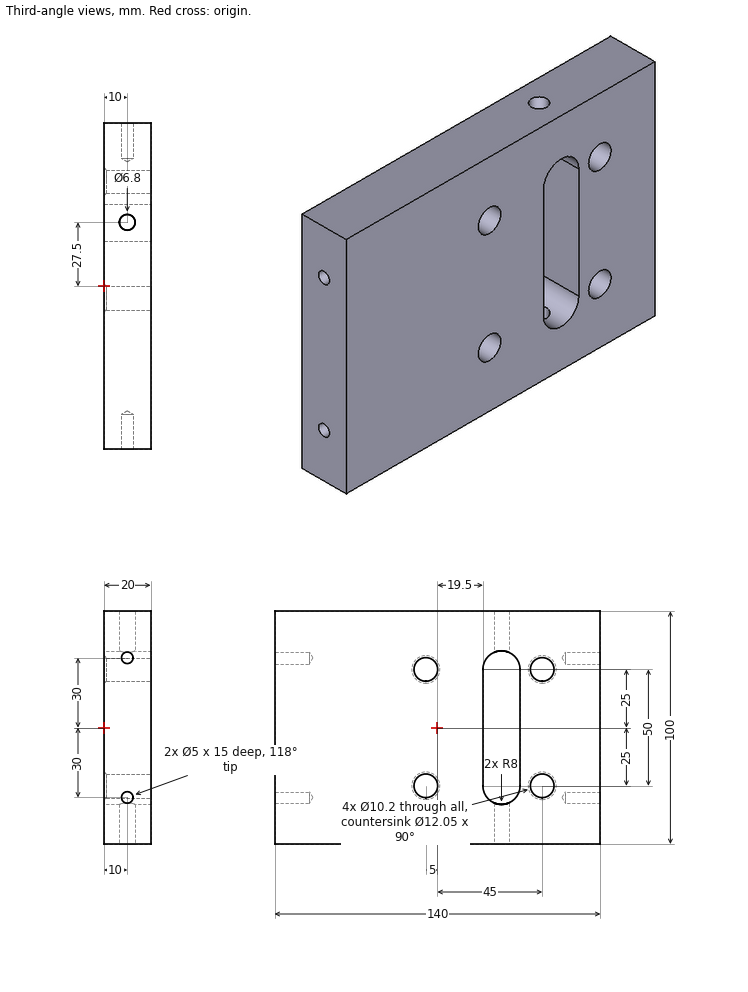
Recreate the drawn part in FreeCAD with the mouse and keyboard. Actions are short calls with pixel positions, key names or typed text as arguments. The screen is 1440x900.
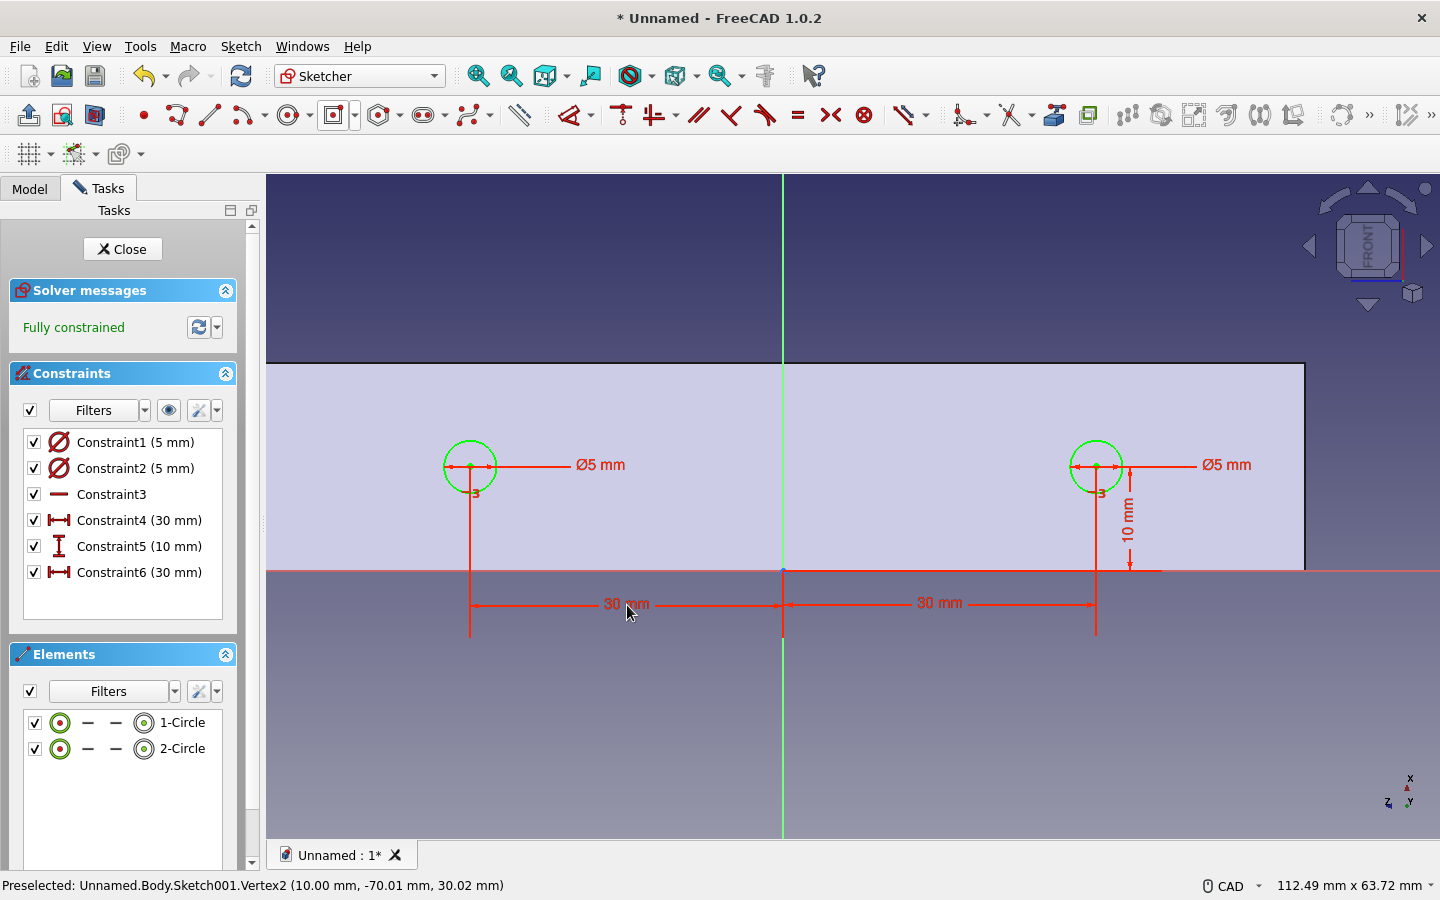
click(123, 249)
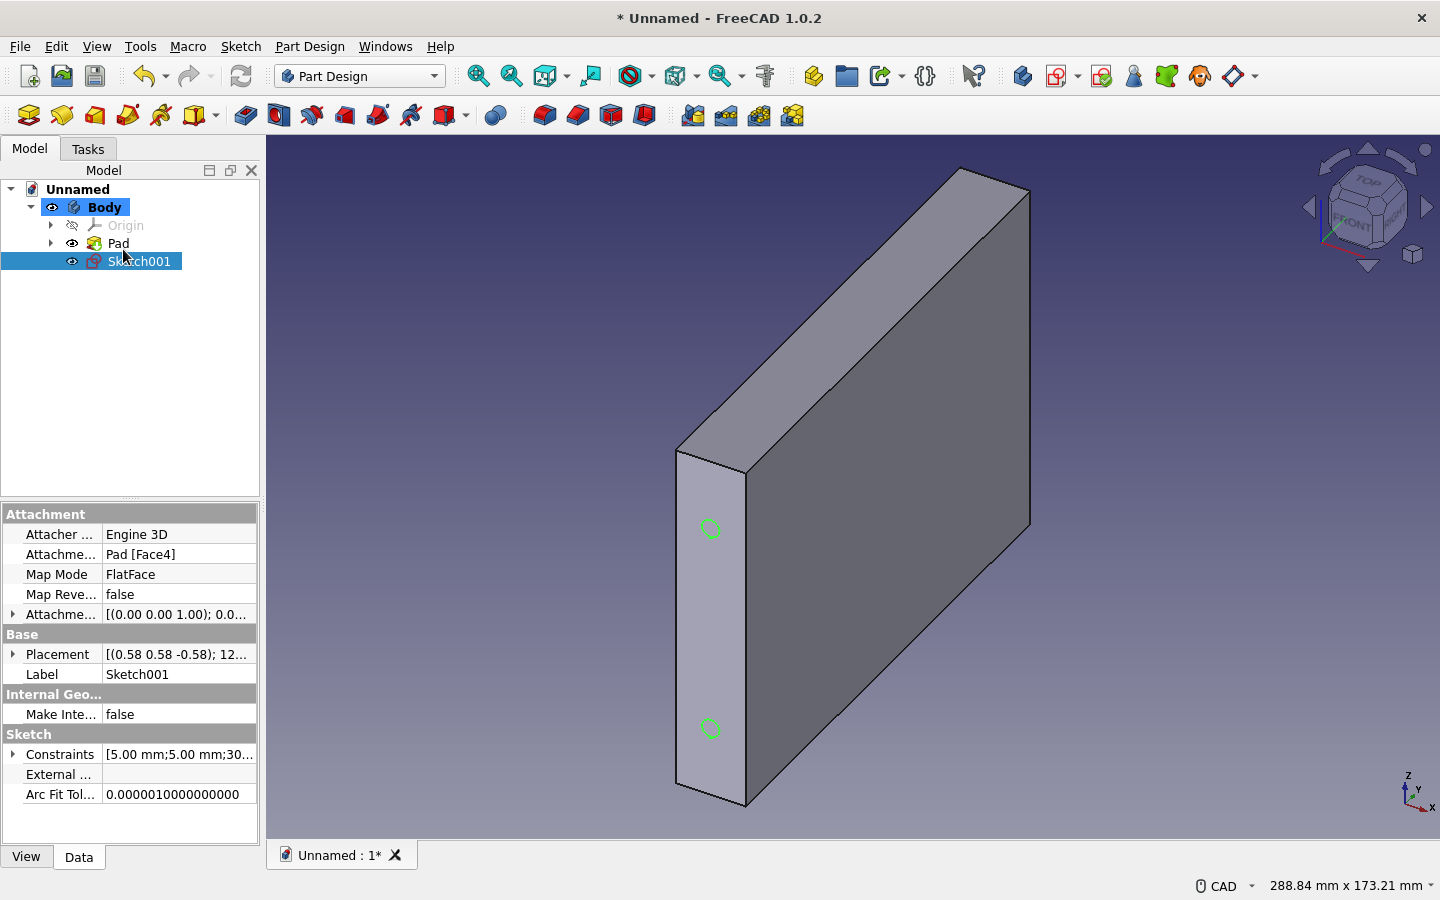
click(279, 116)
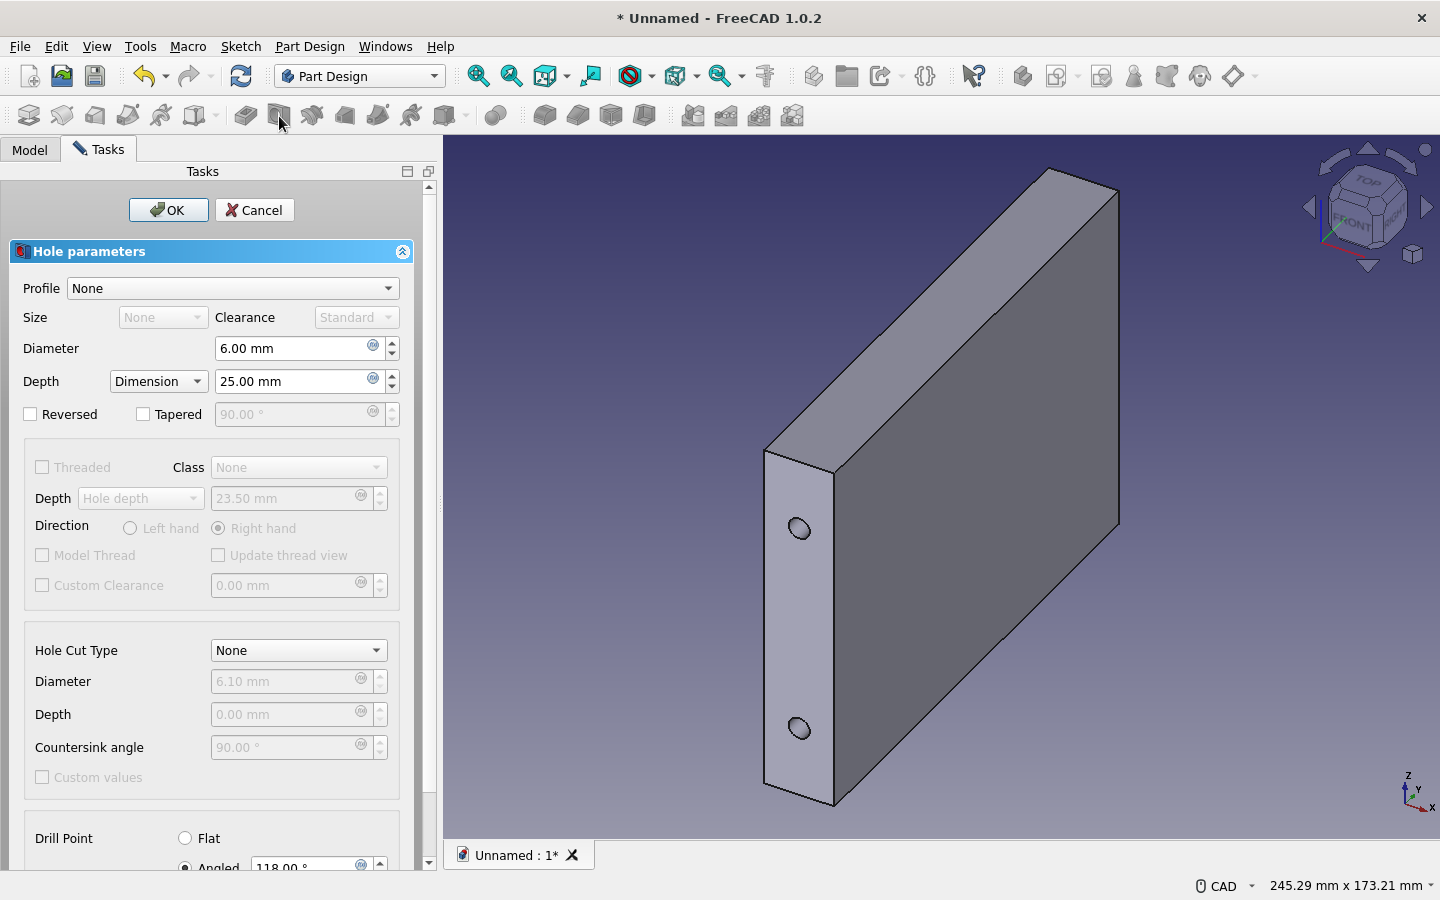
triple_click(300, 348)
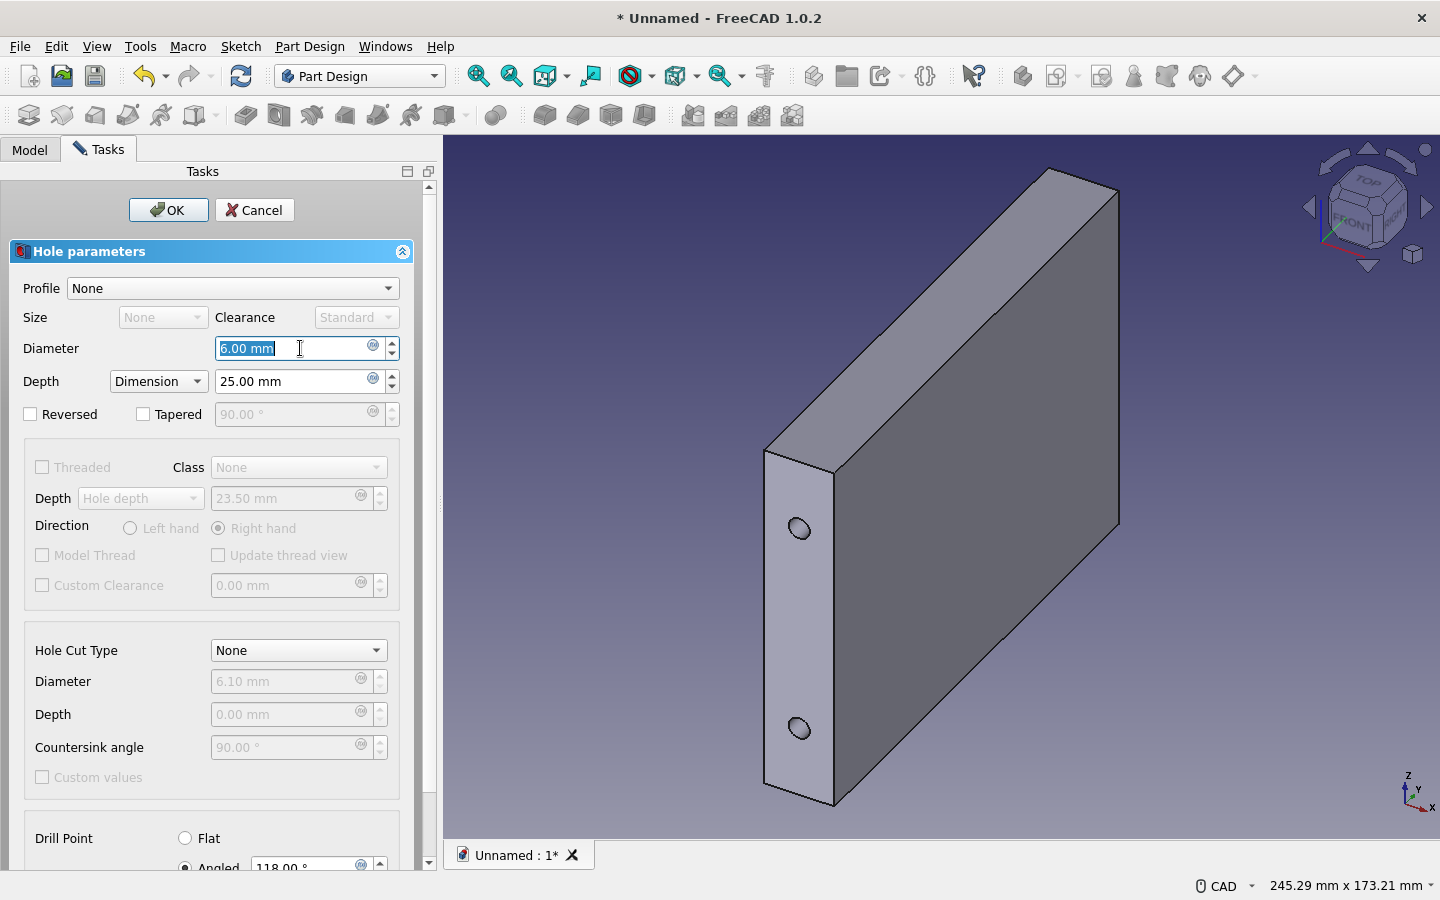
text(5)
key(Tab)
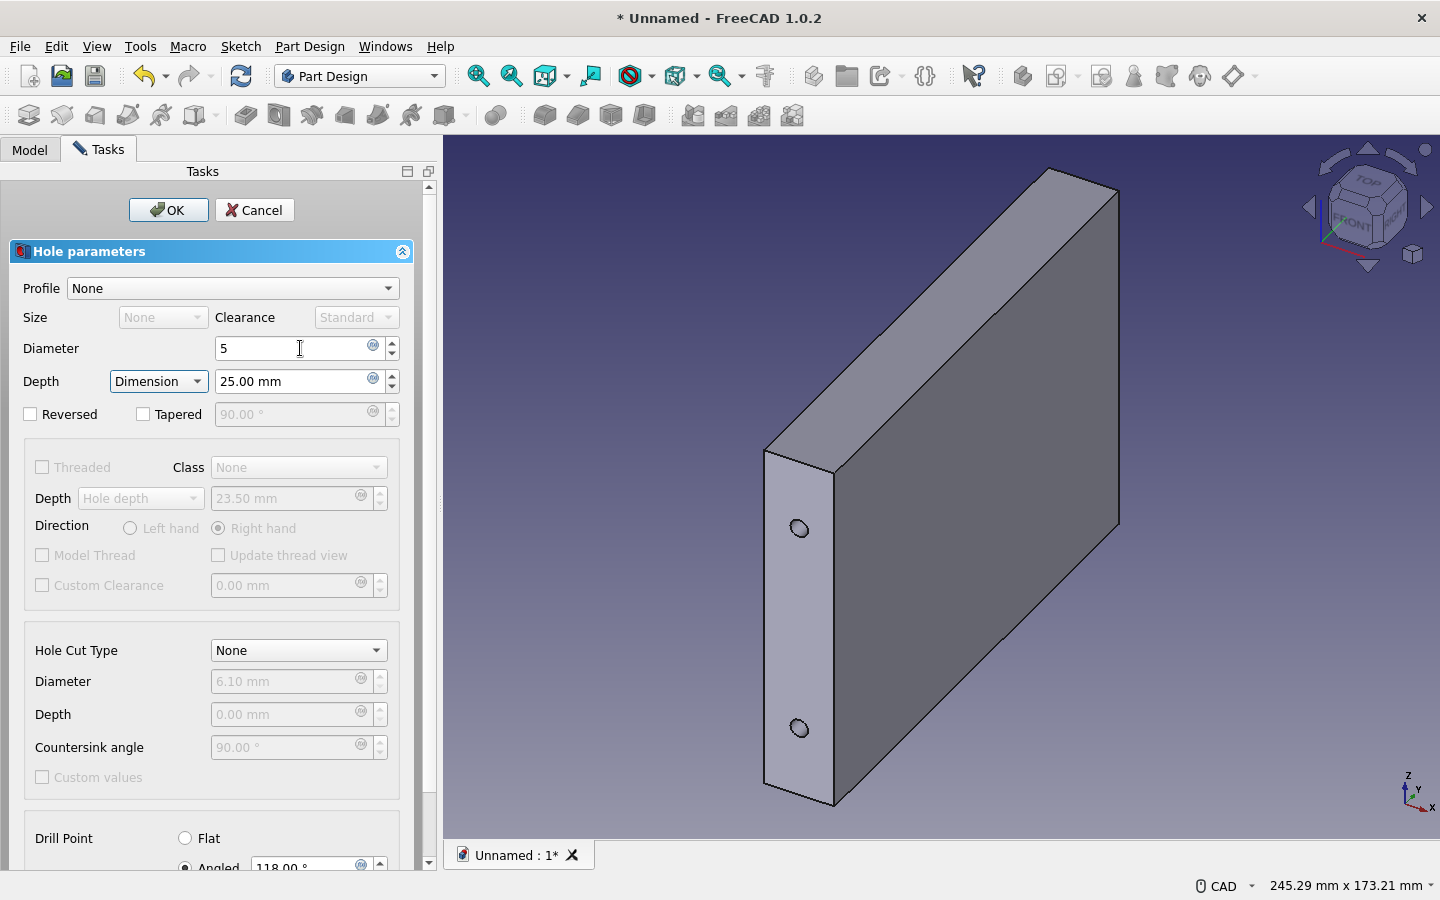
triple_click(300, 382)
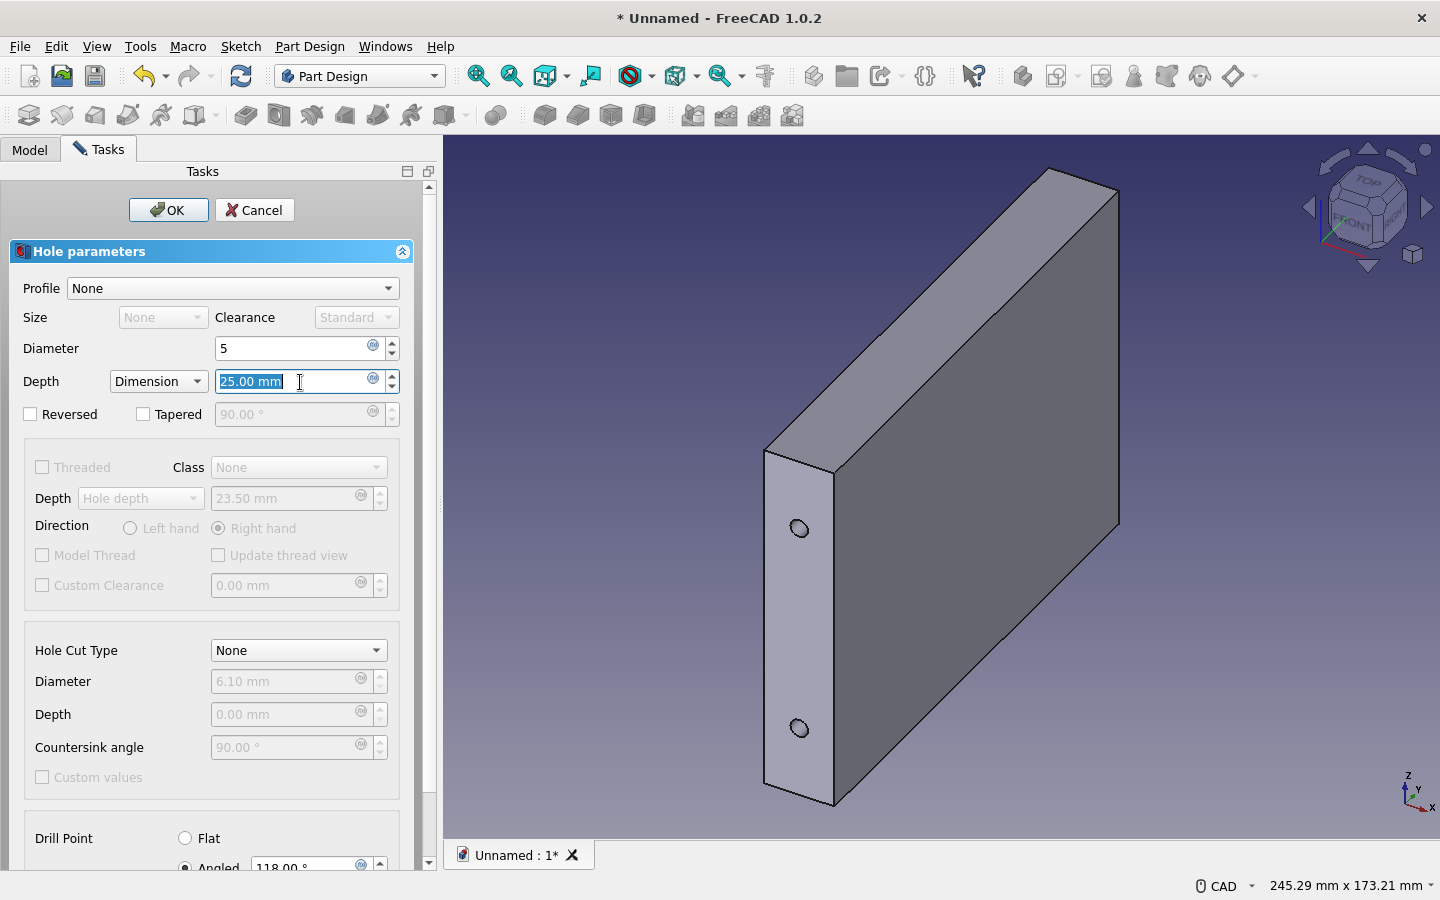
text(15)
key(Tab)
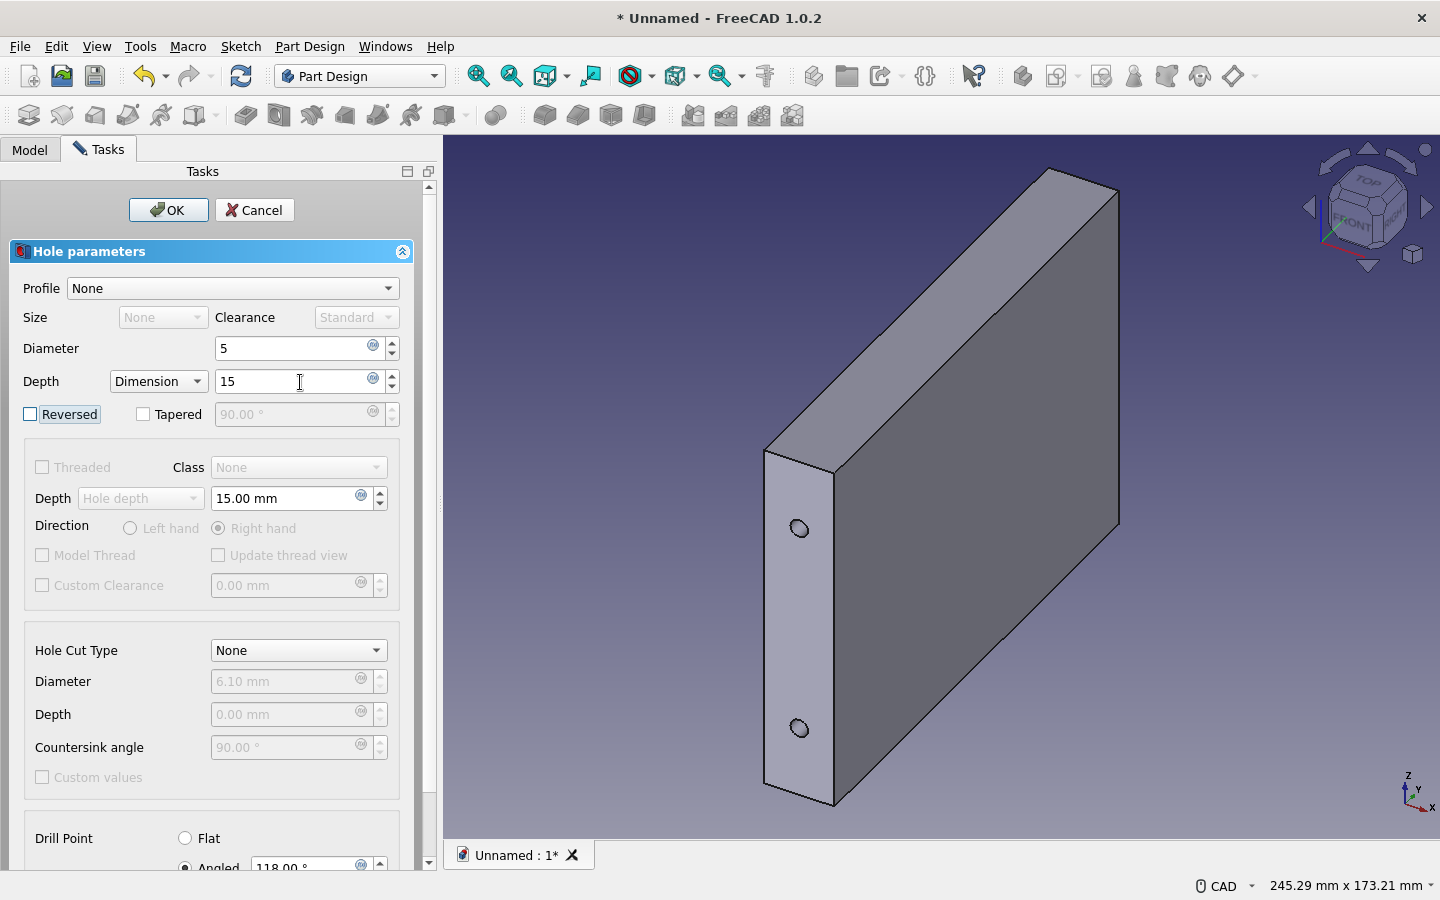
click(169, 210)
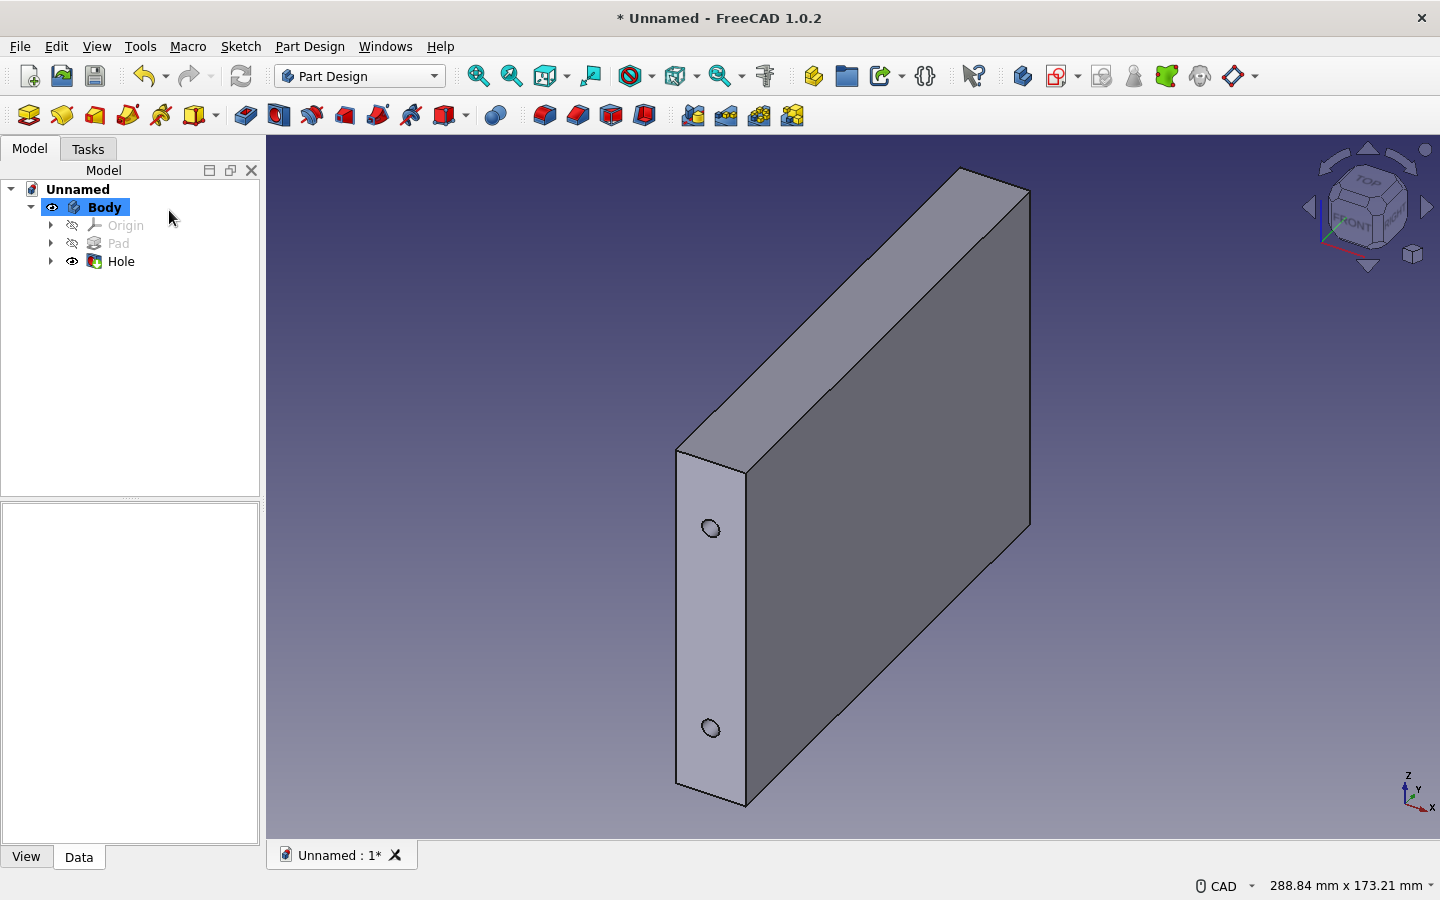
key(6)